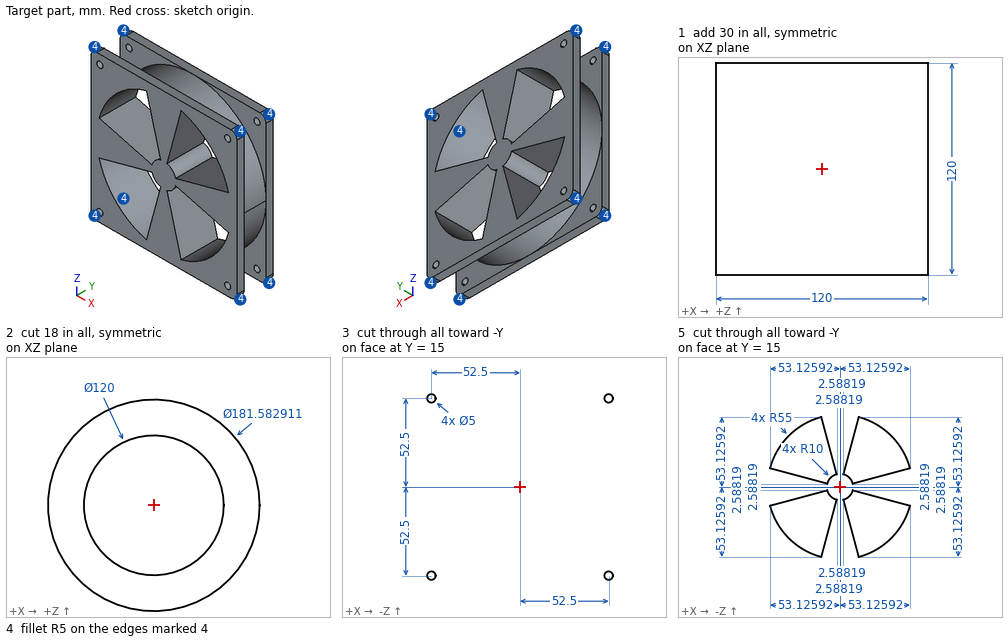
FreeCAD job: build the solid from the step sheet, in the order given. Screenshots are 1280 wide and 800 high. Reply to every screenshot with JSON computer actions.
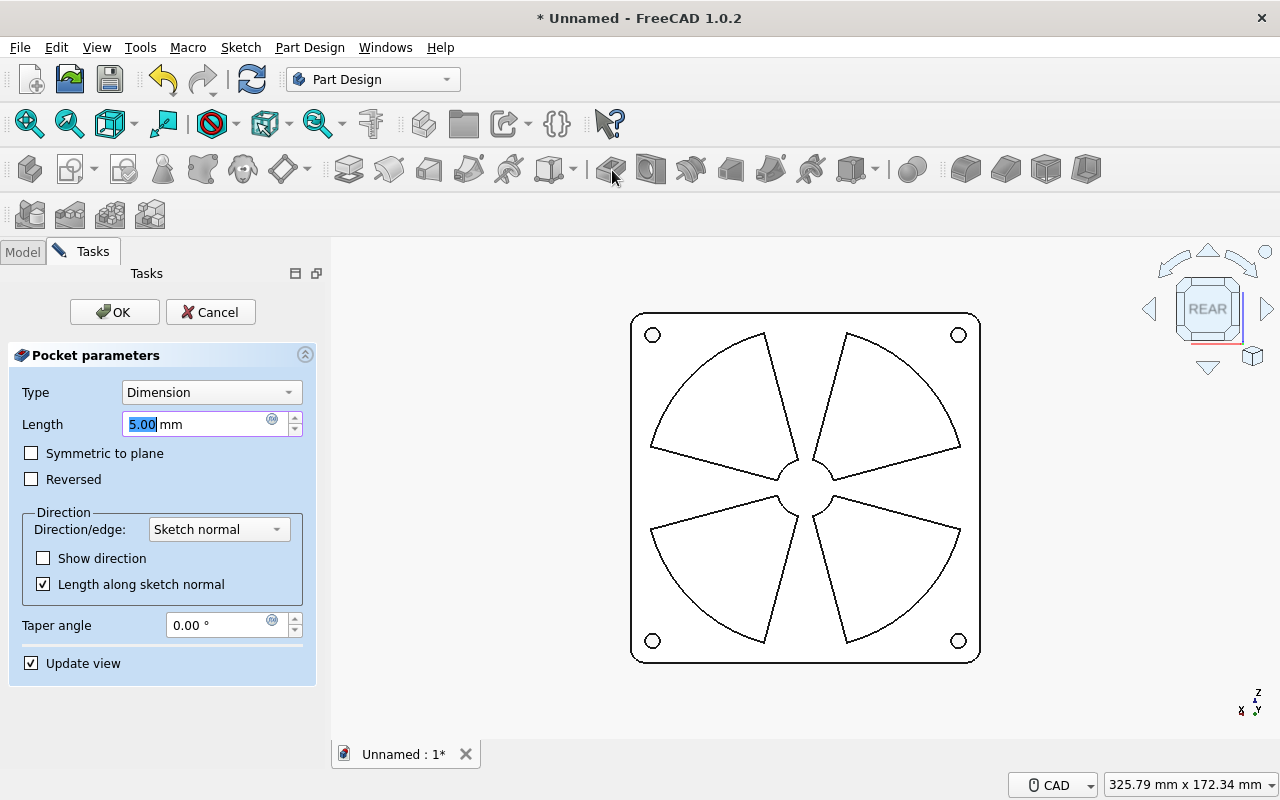
{"action": "left_click", "coordinate": [212, 392]}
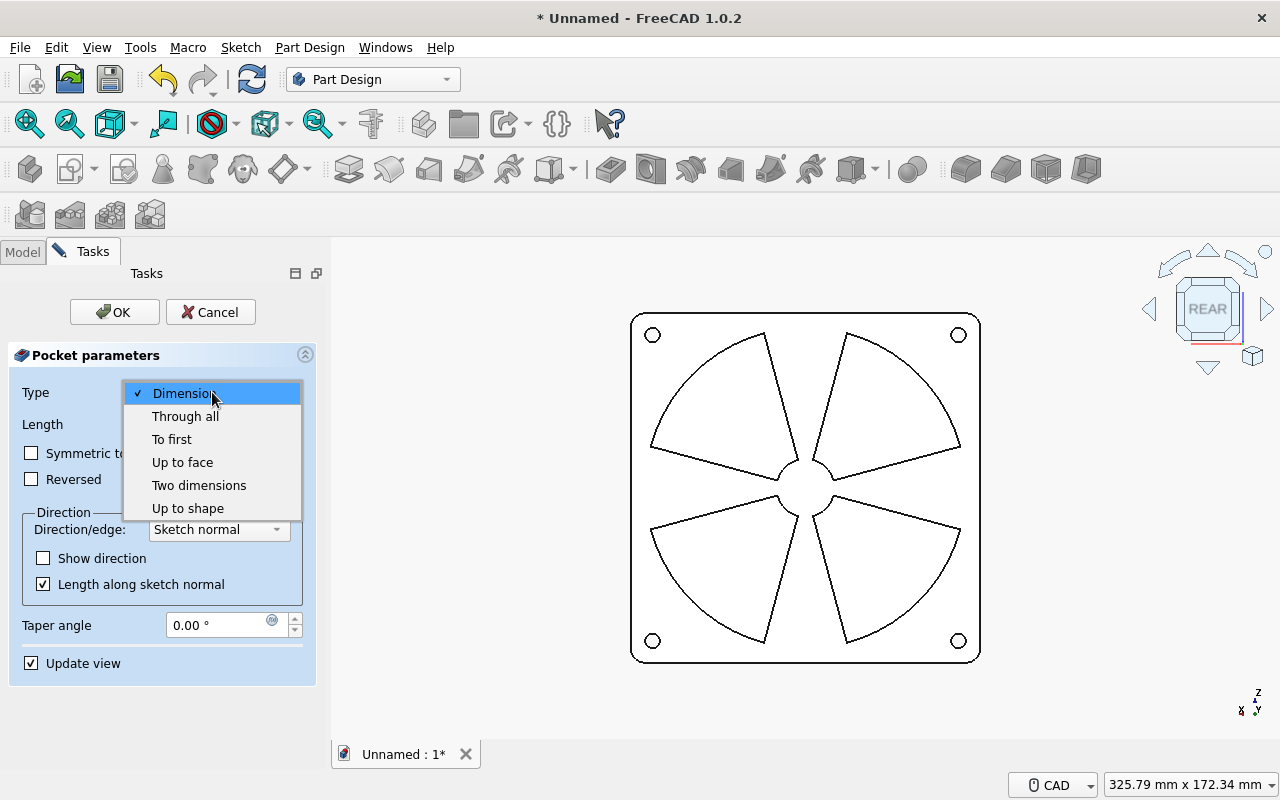
{"action": "left_click", "coordinate": [212, 416]}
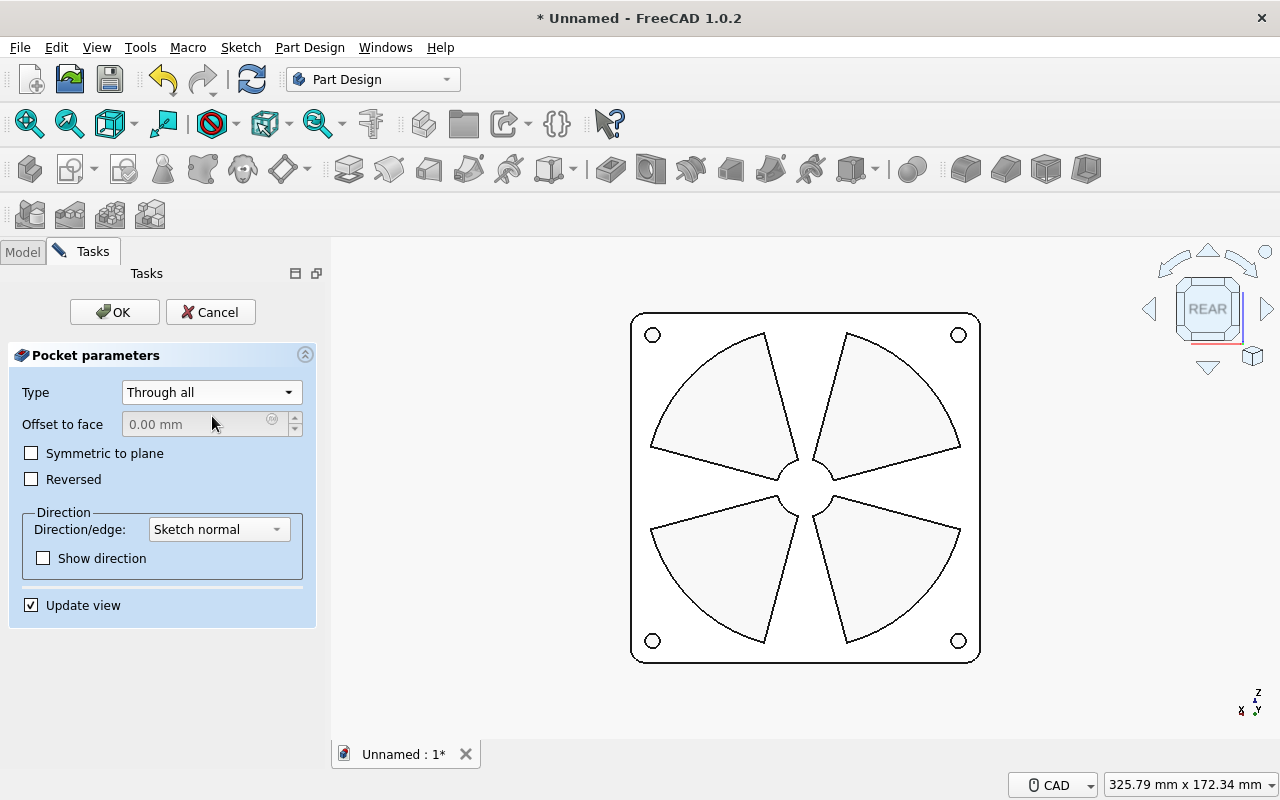
{"action": "left_click", "coordinate": [115, 312]}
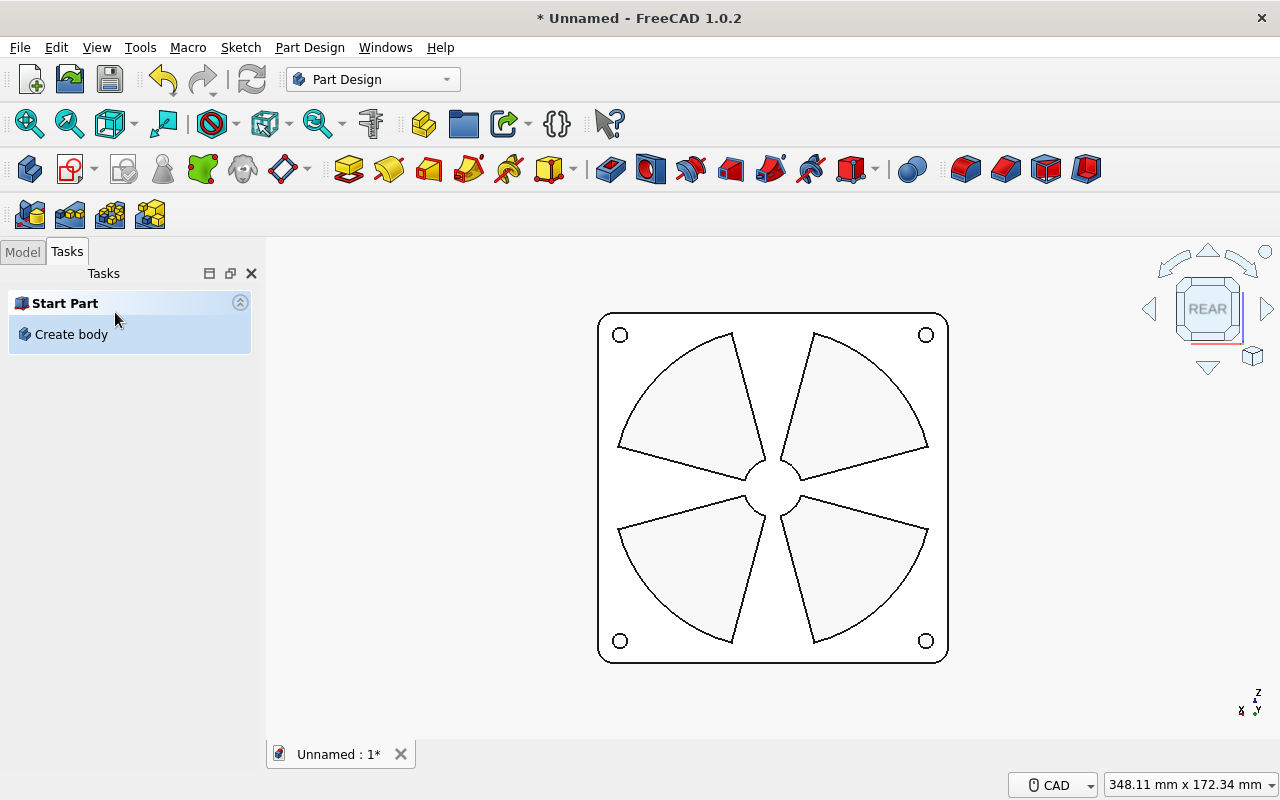
{"action": "key", "text": "0"}